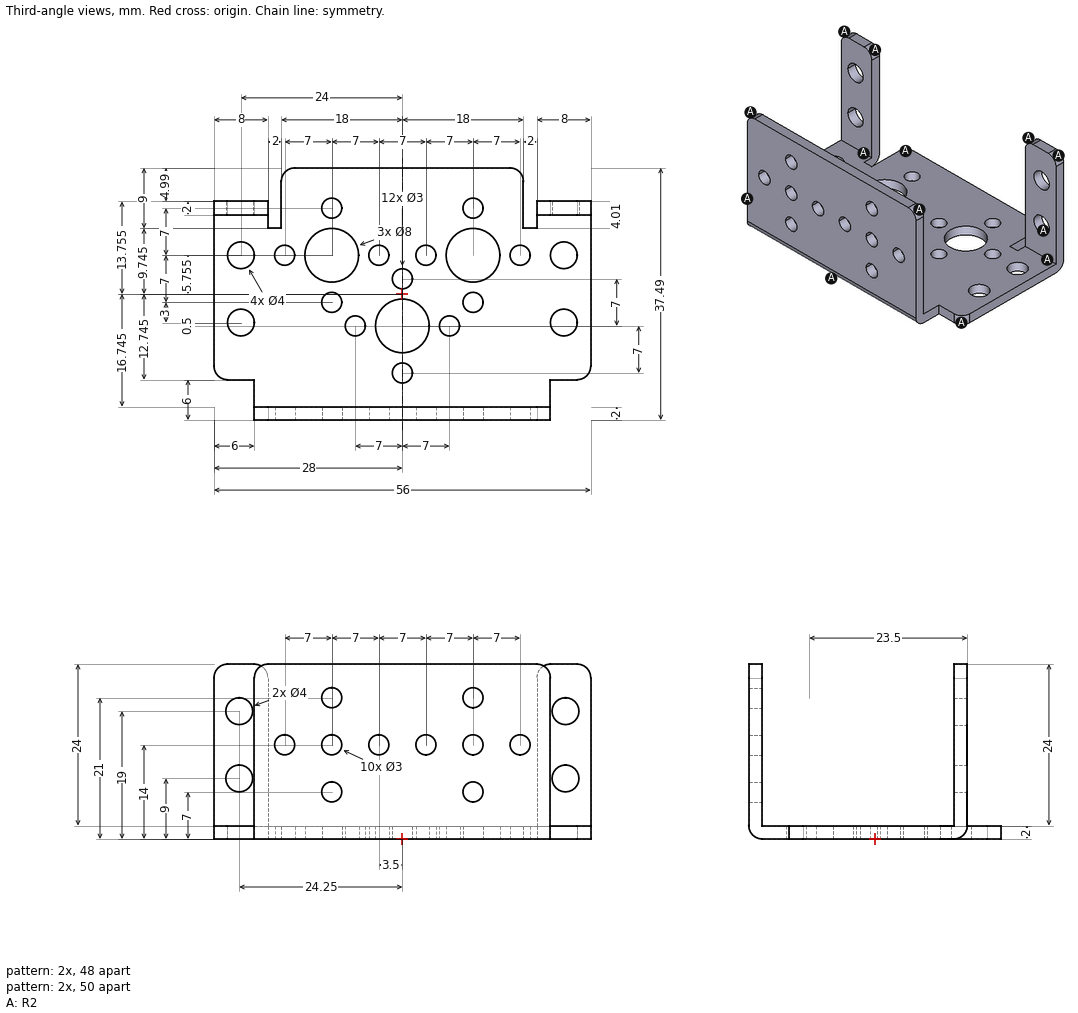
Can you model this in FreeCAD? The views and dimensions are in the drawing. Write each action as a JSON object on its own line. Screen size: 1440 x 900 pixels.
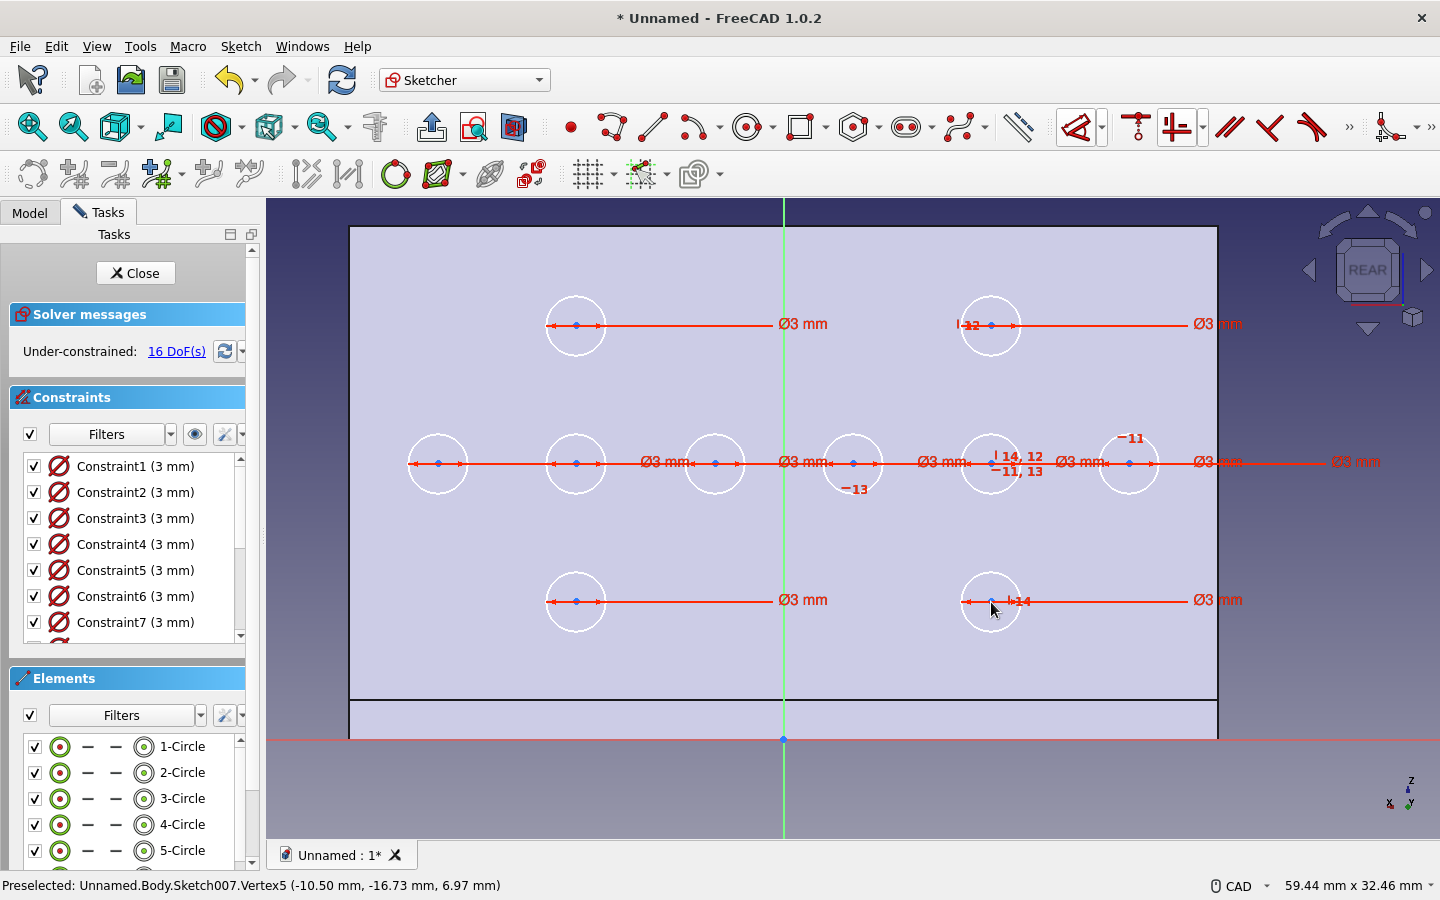
{"action": "left_click", "coordinate": [991, 326]}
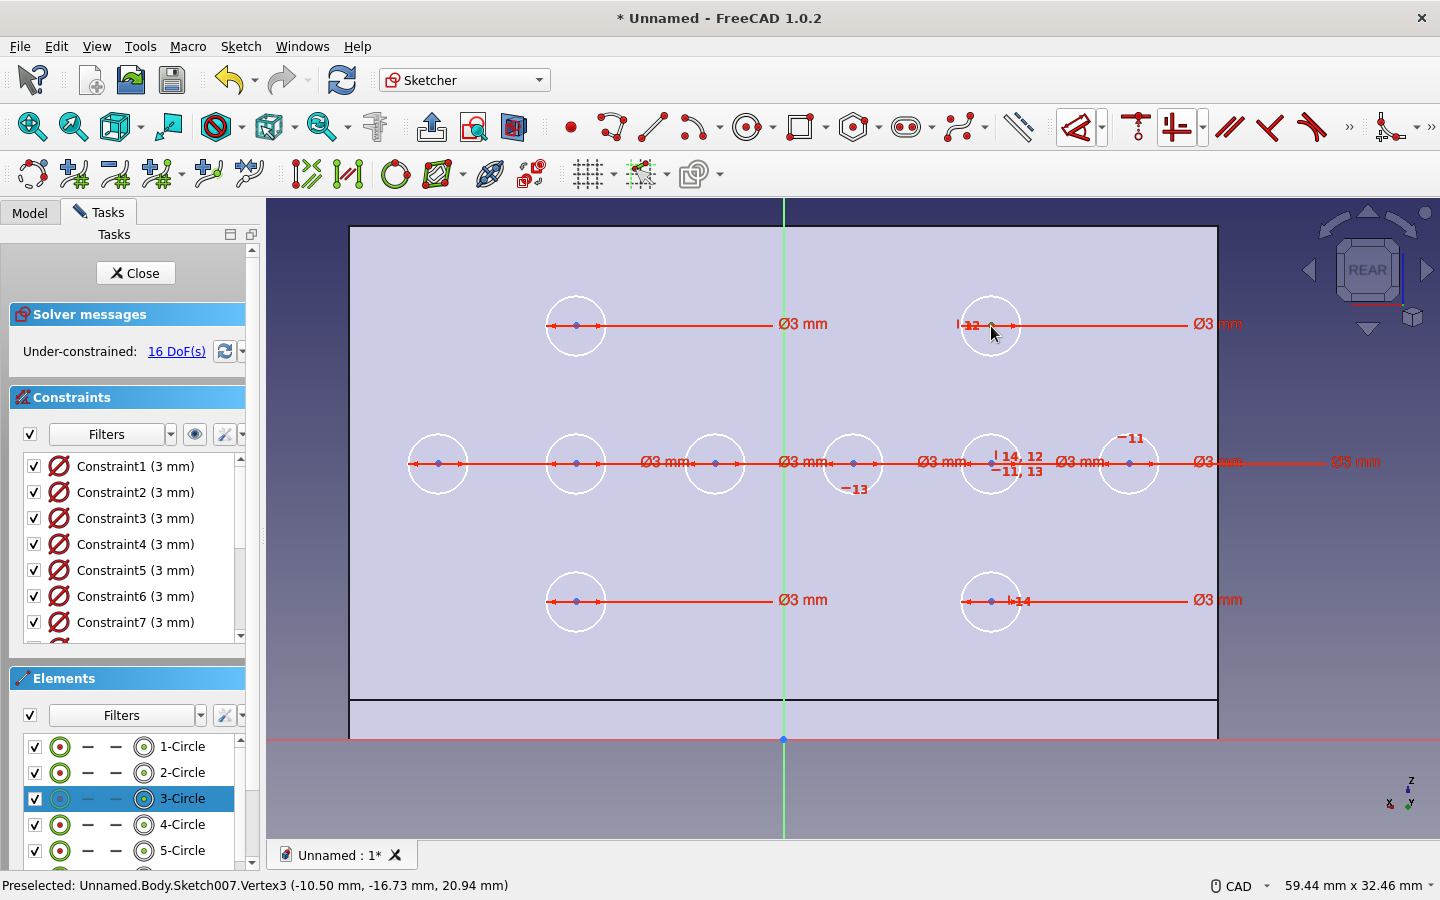
{"action": "left_click", "coordinate": [576, 326]}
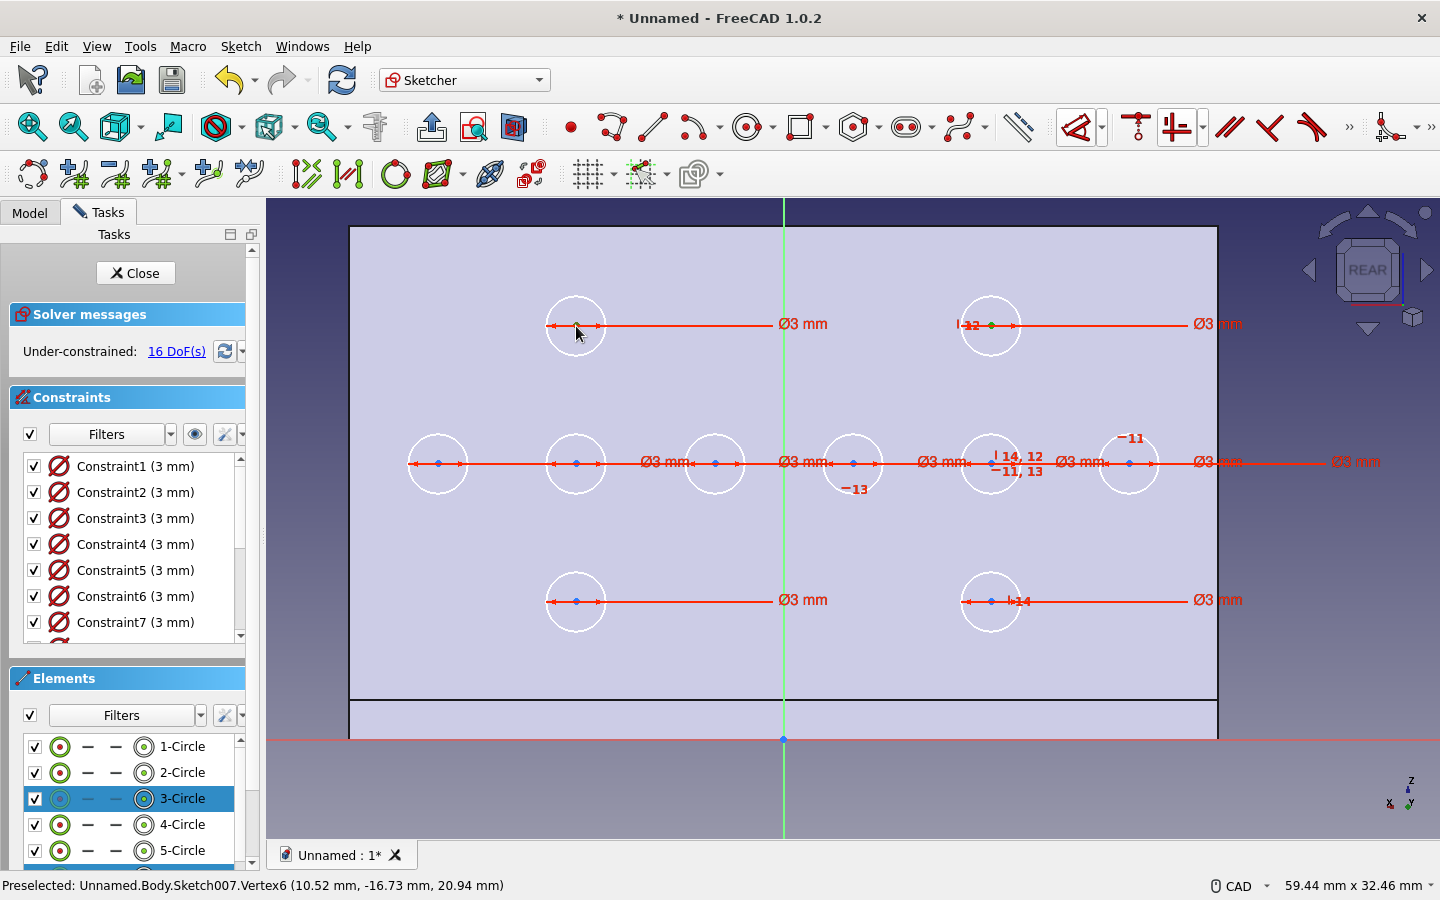
{"action": "key", "text": "h"}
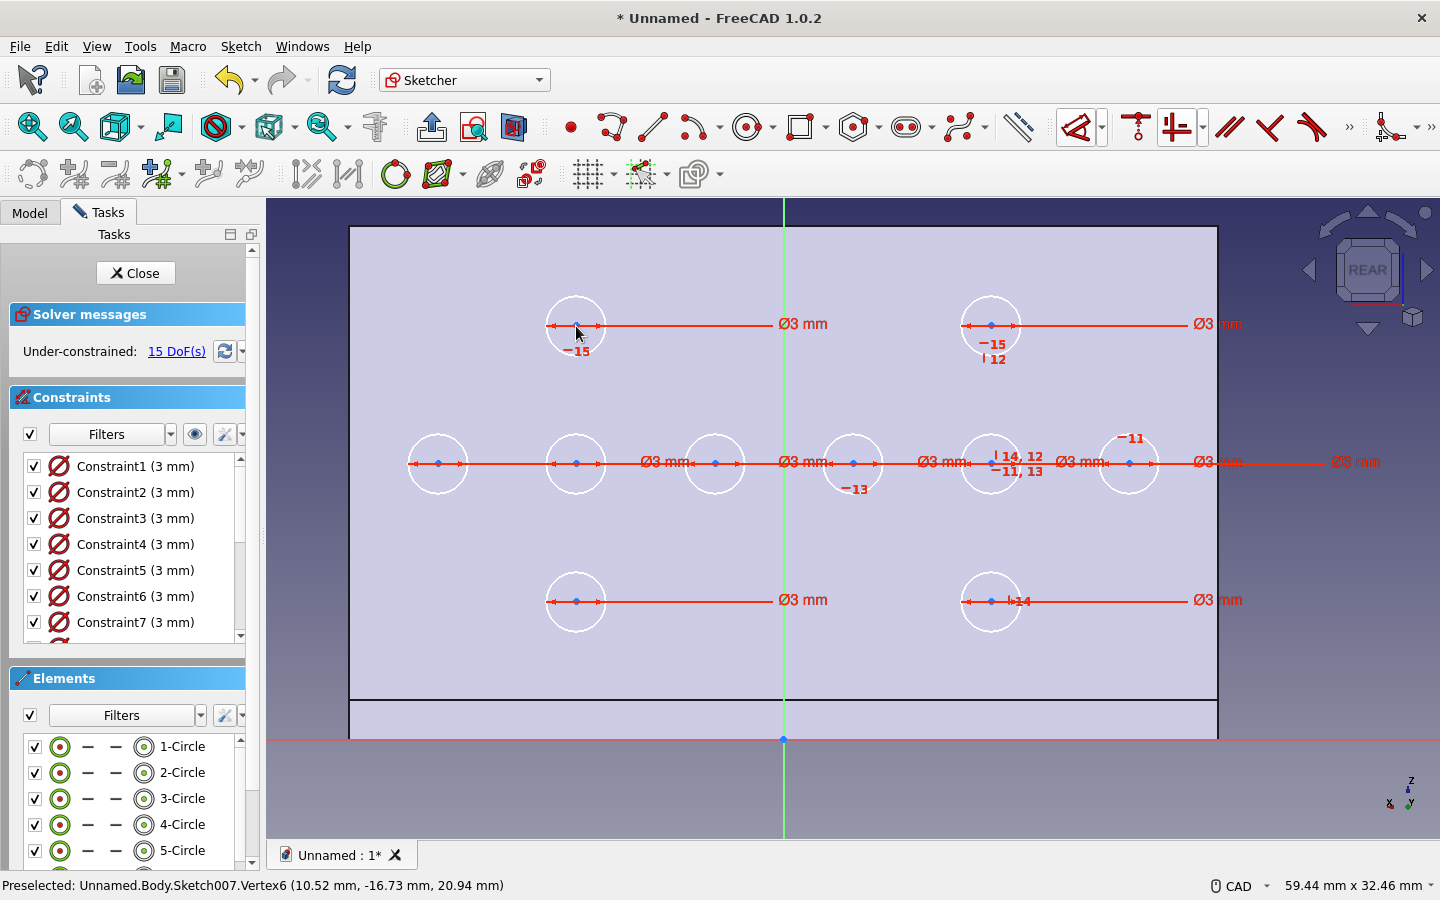
{"action": "left_click", "coordinate": [853, 464]}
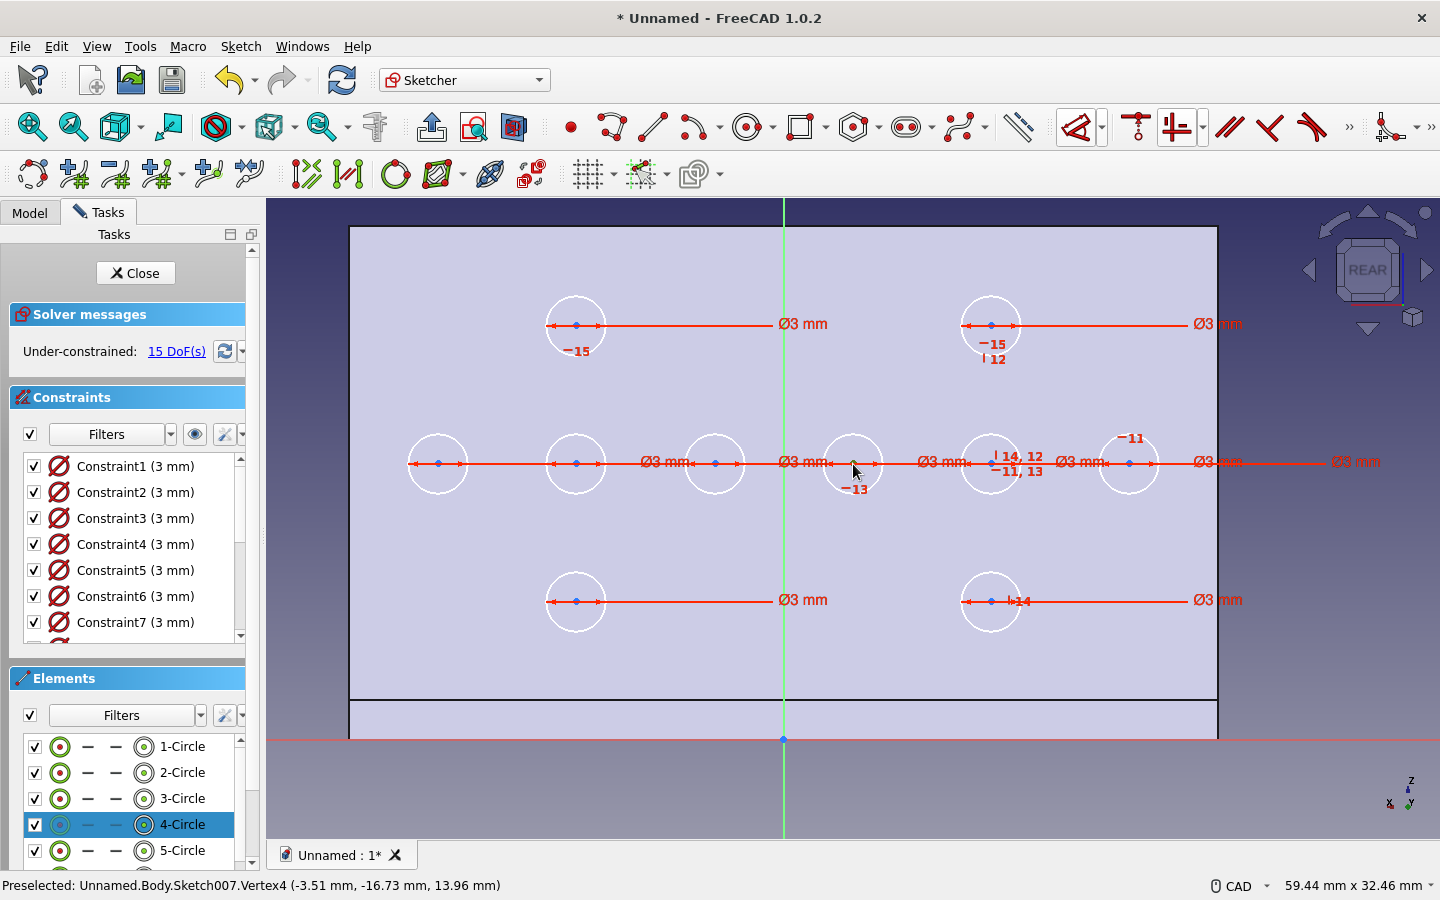
{"action": "left_click", "coordinate": [715, 464]}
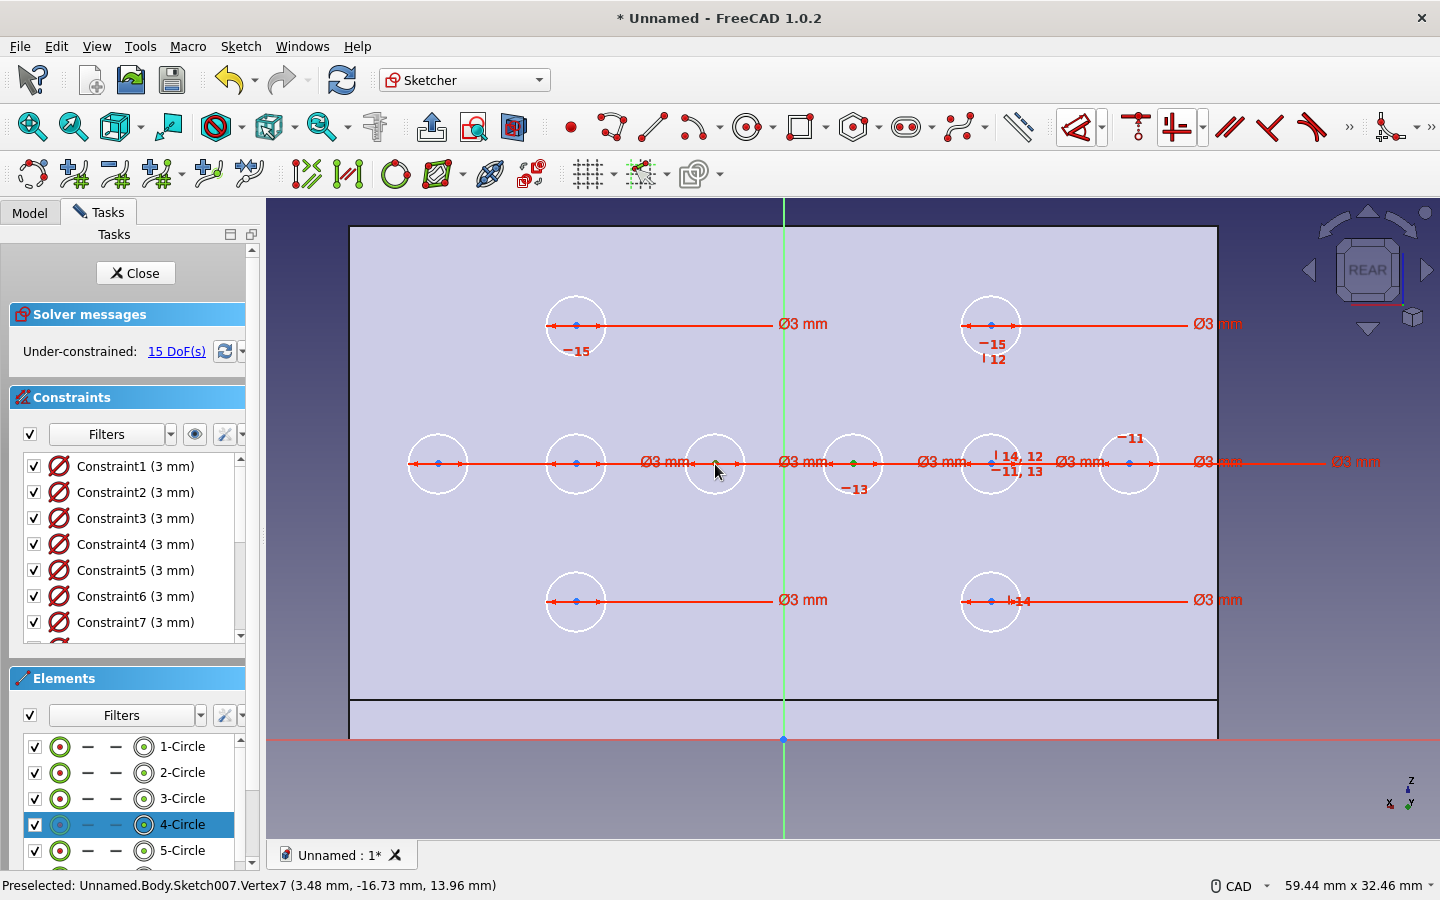
{"action": "key", "text": "h"}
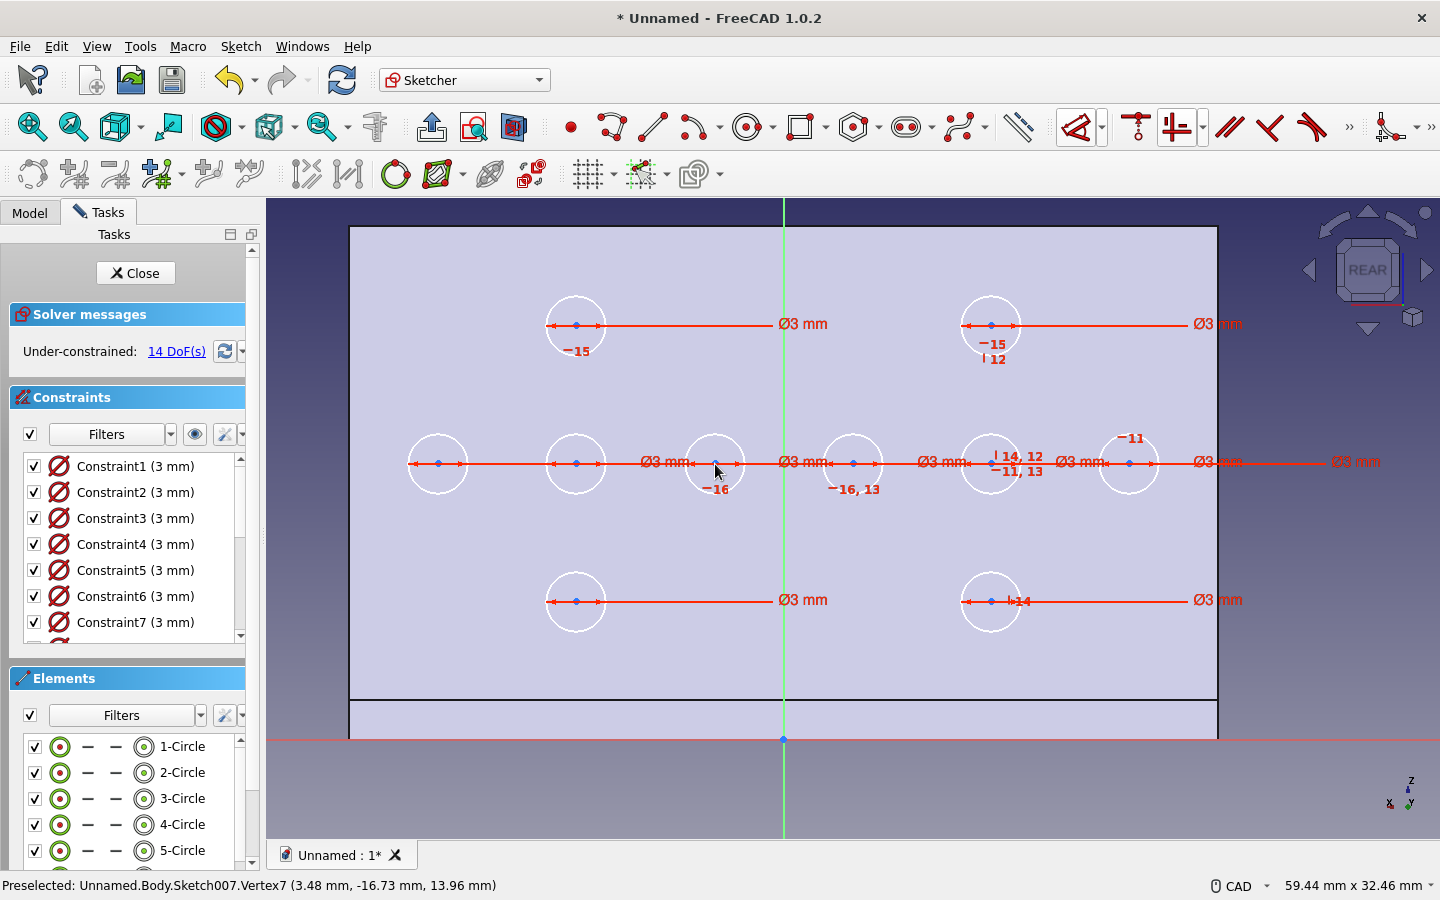
{"action": "left_click", "coordinate": [576, 326]}